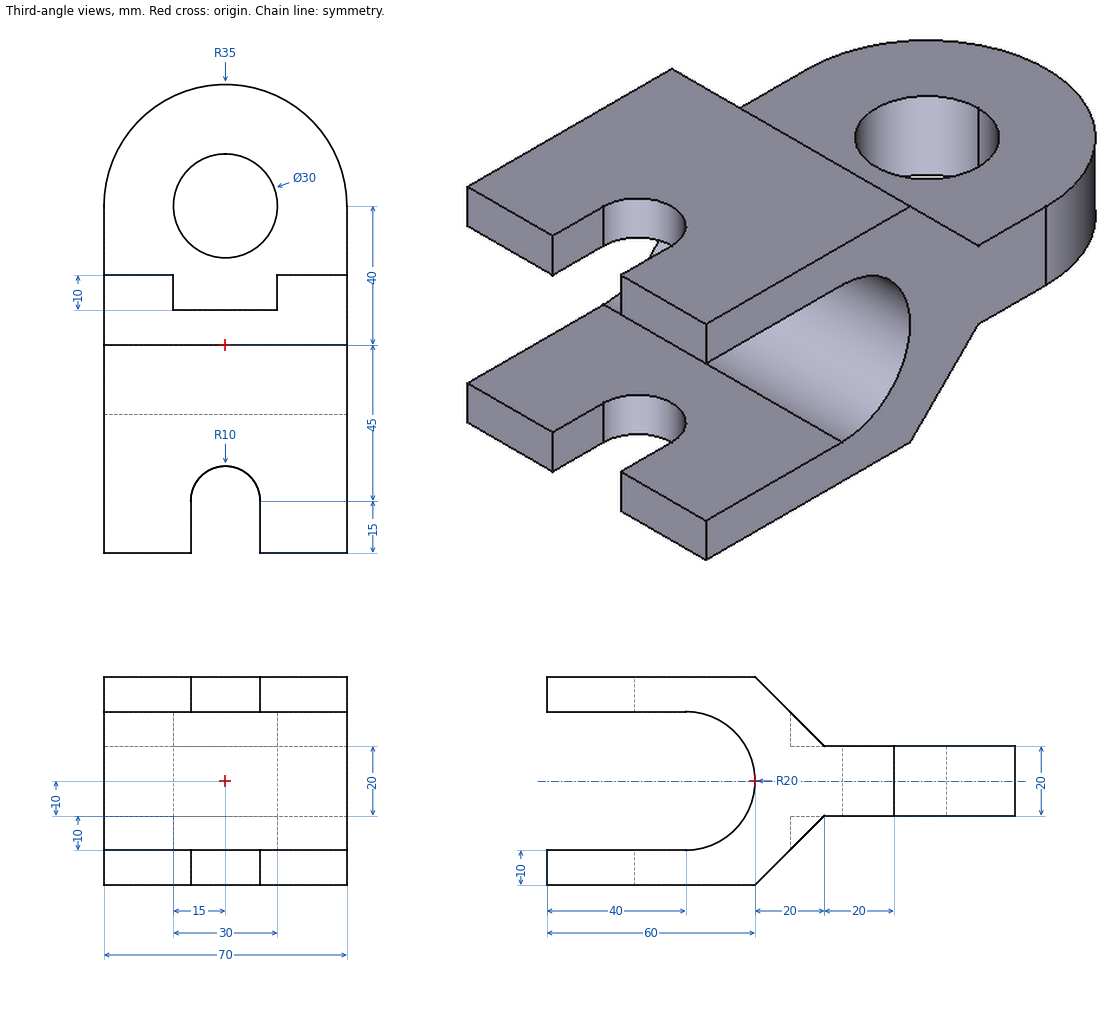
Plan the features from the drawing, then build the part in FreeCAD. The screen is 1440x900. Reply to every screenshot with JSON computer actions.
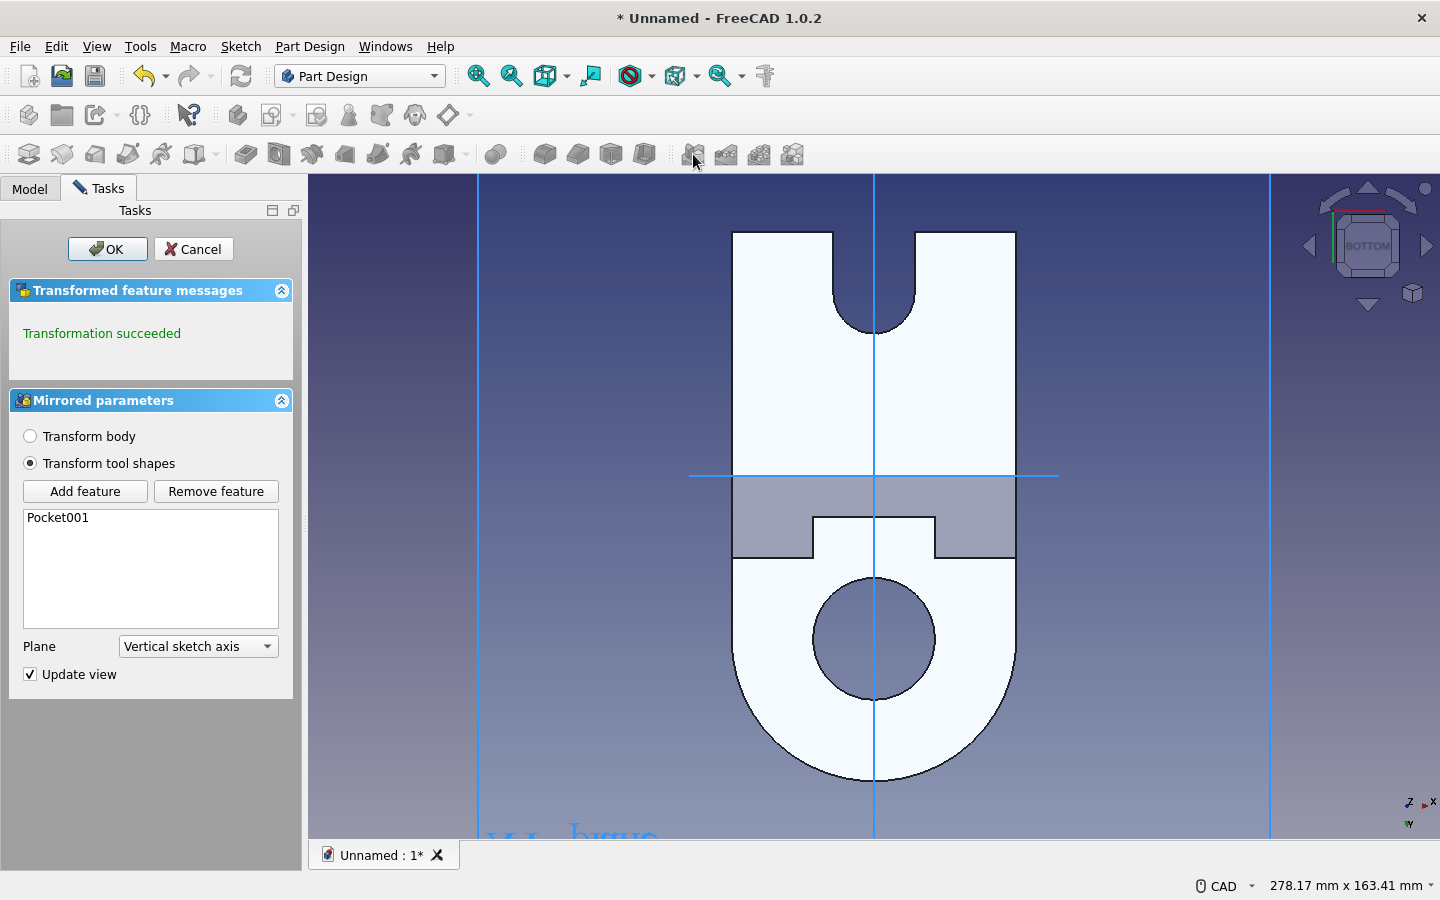
{"action": "left_click", "coordinate": [199, 646]}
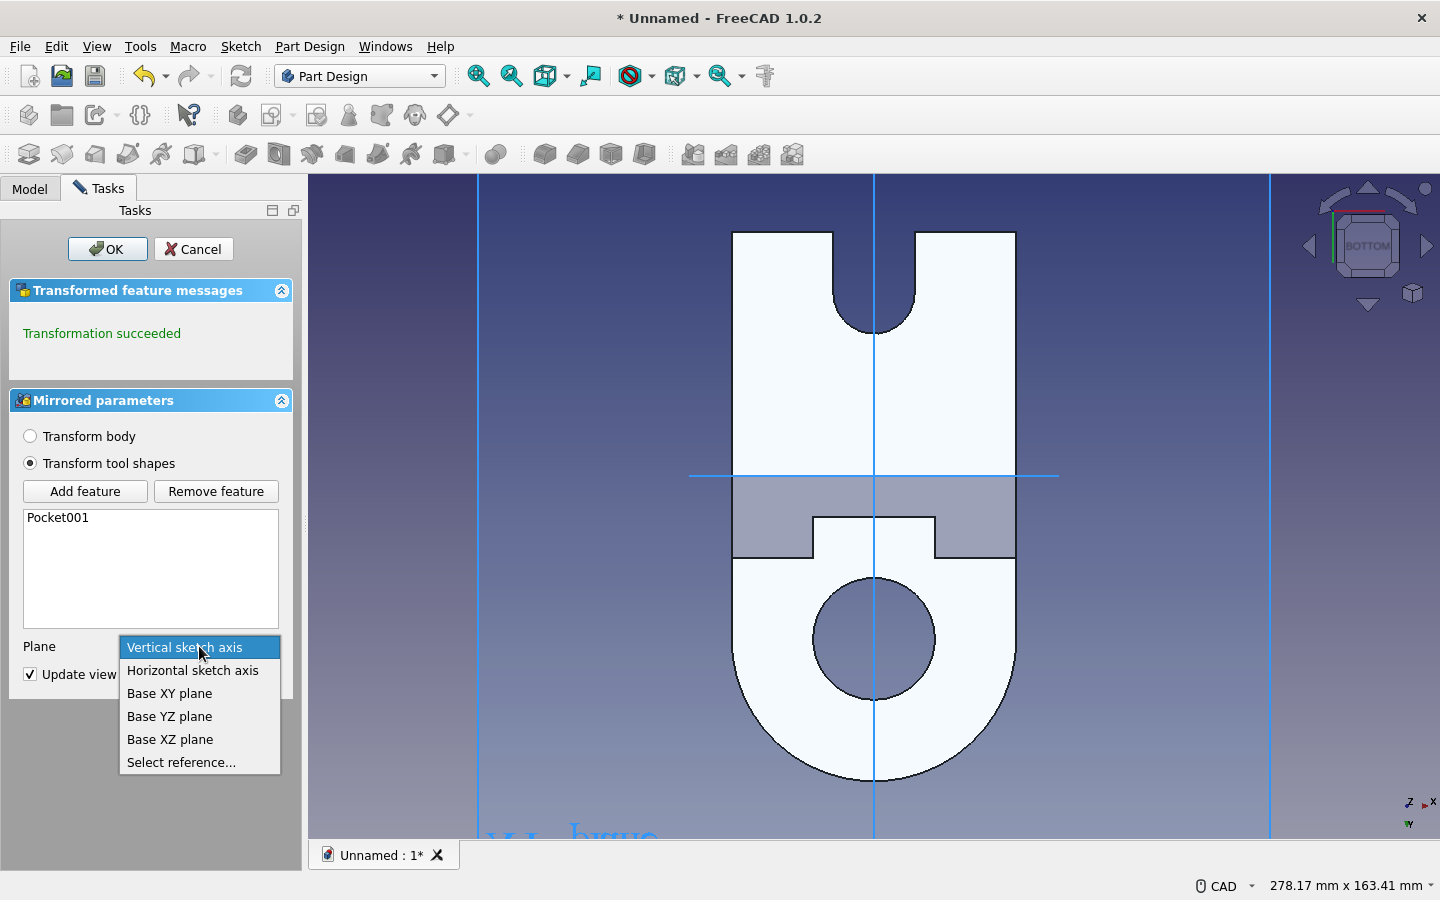
{"action": "left_click", "coordinate": [198, 694]}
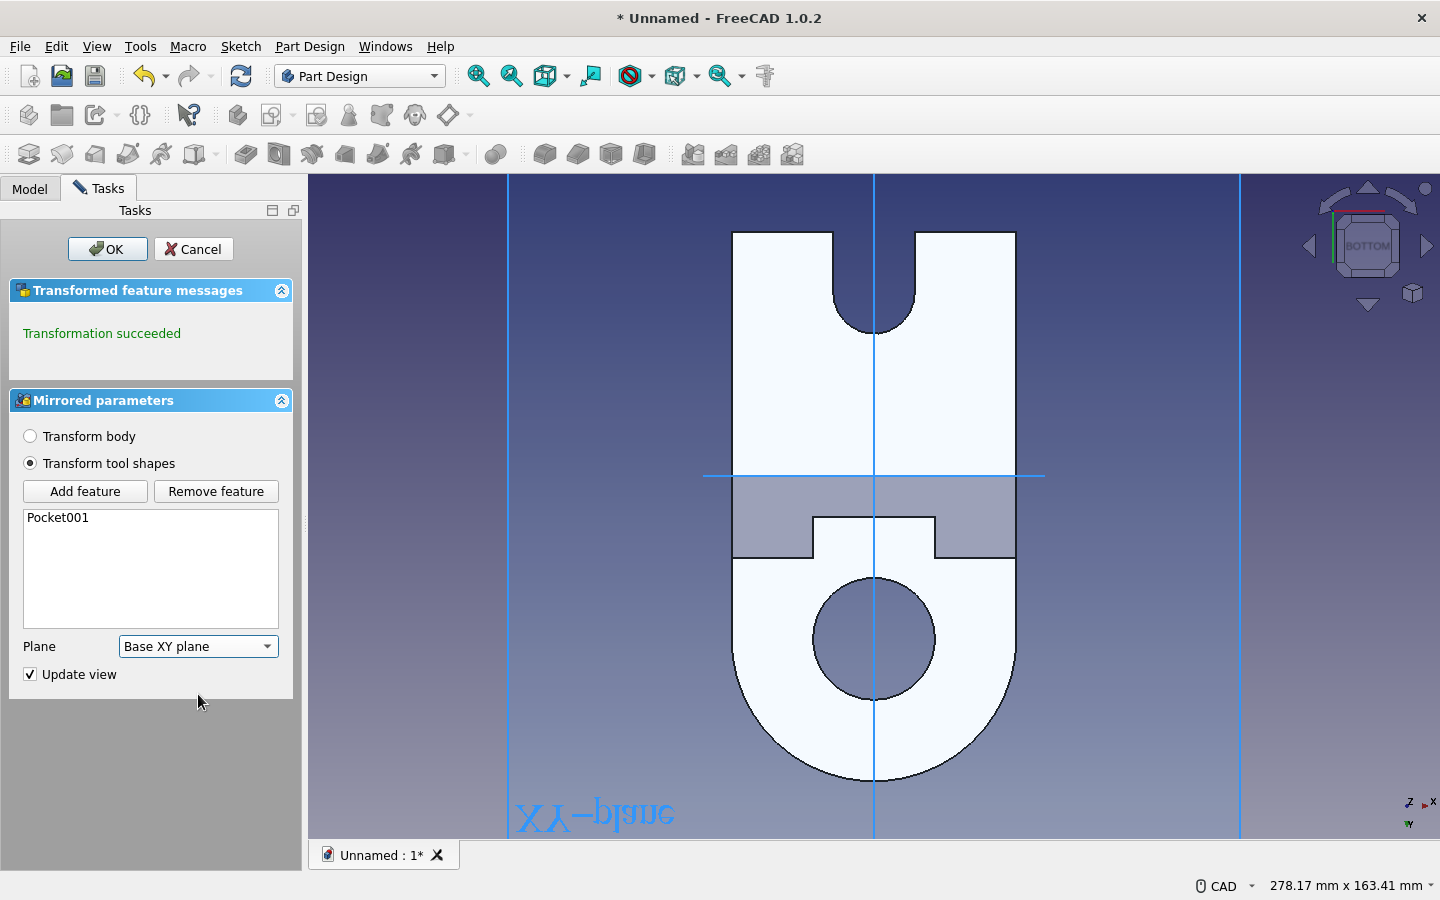
{"action": "left_click", "coordinate": [108, 249]}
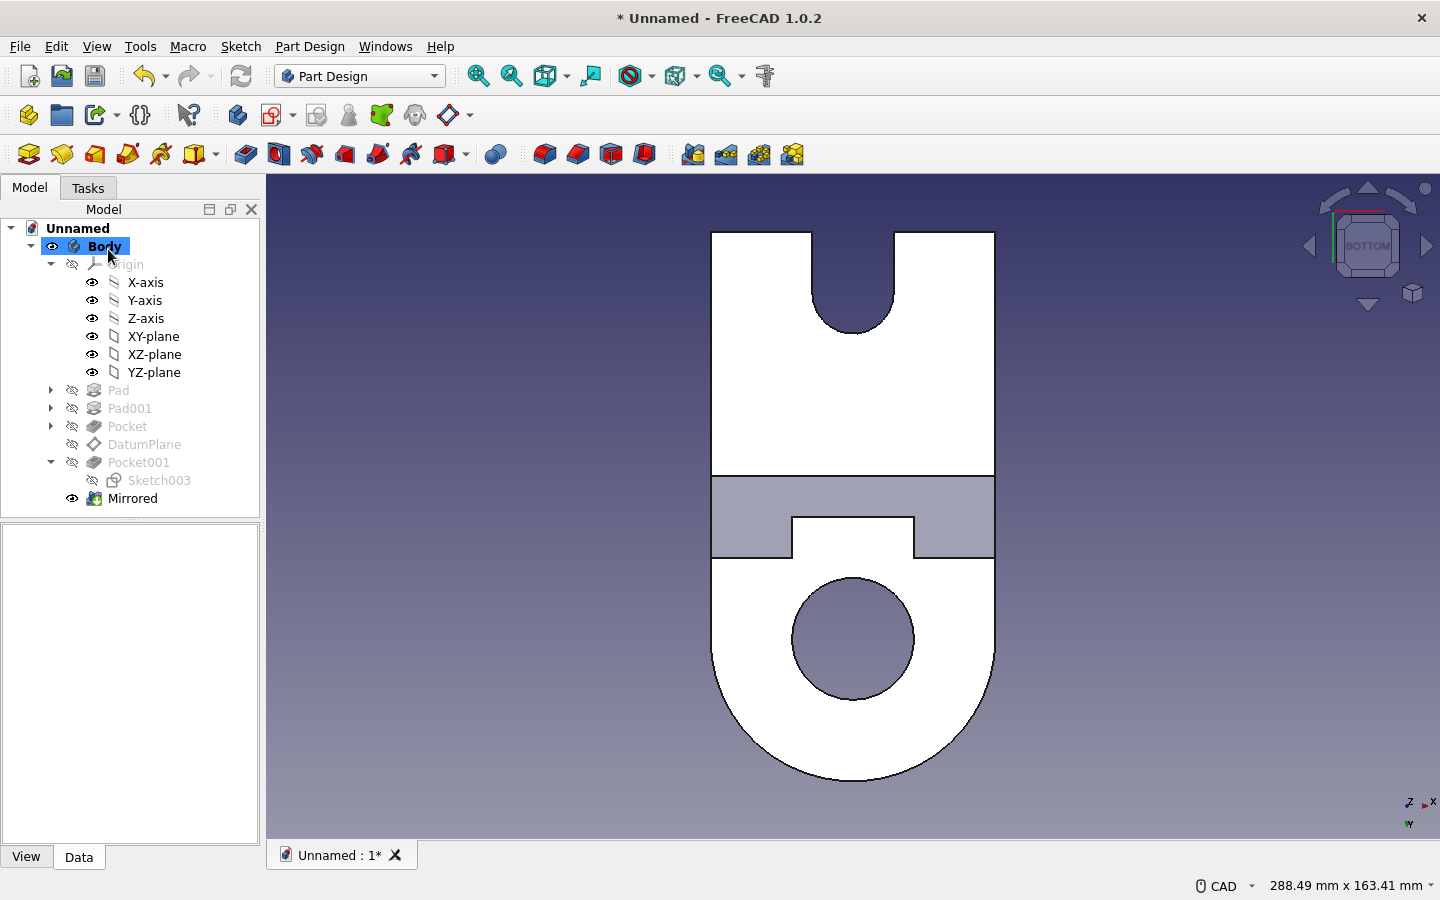
{"action": "key", "text": "0"}